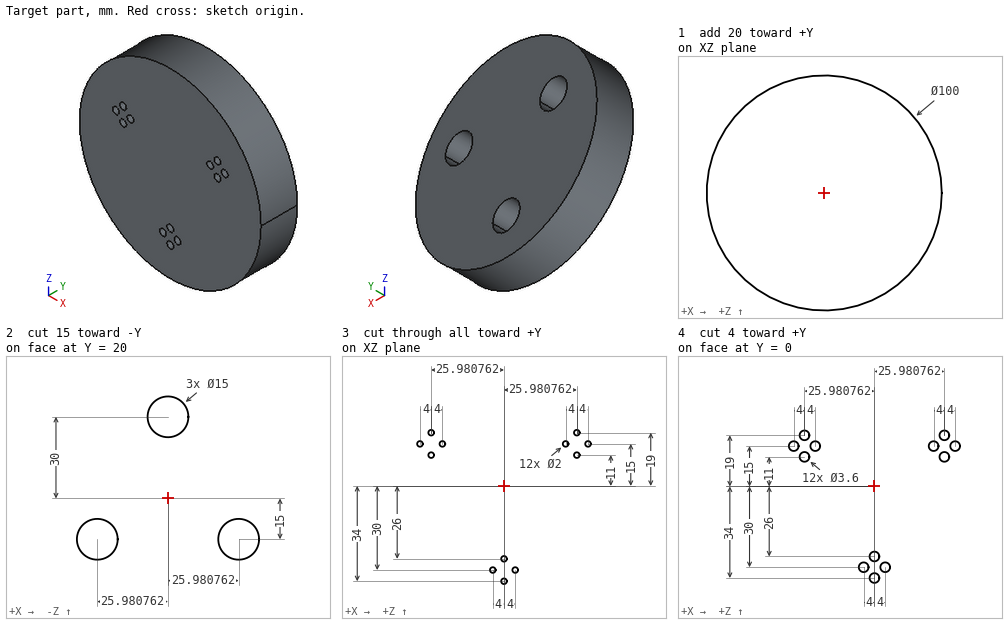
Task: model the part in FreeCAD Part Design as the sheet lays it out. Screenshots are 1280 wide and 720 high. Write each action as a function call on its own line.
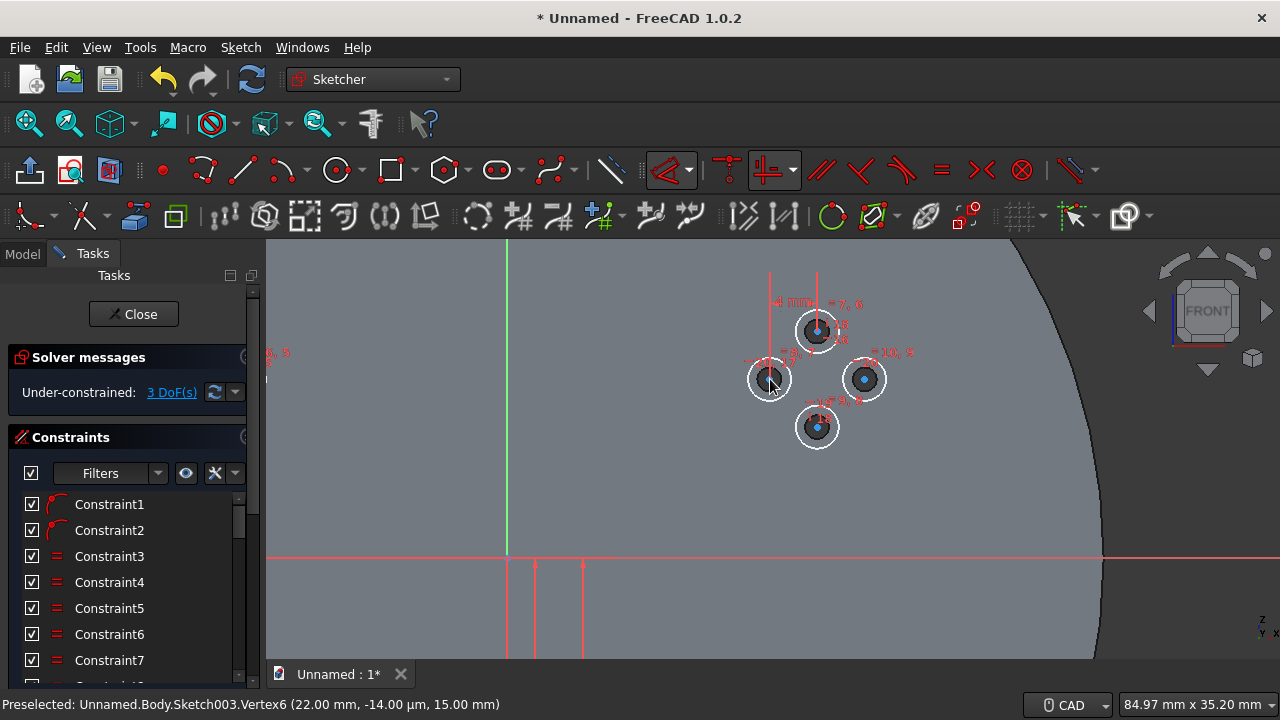
click(817, 332)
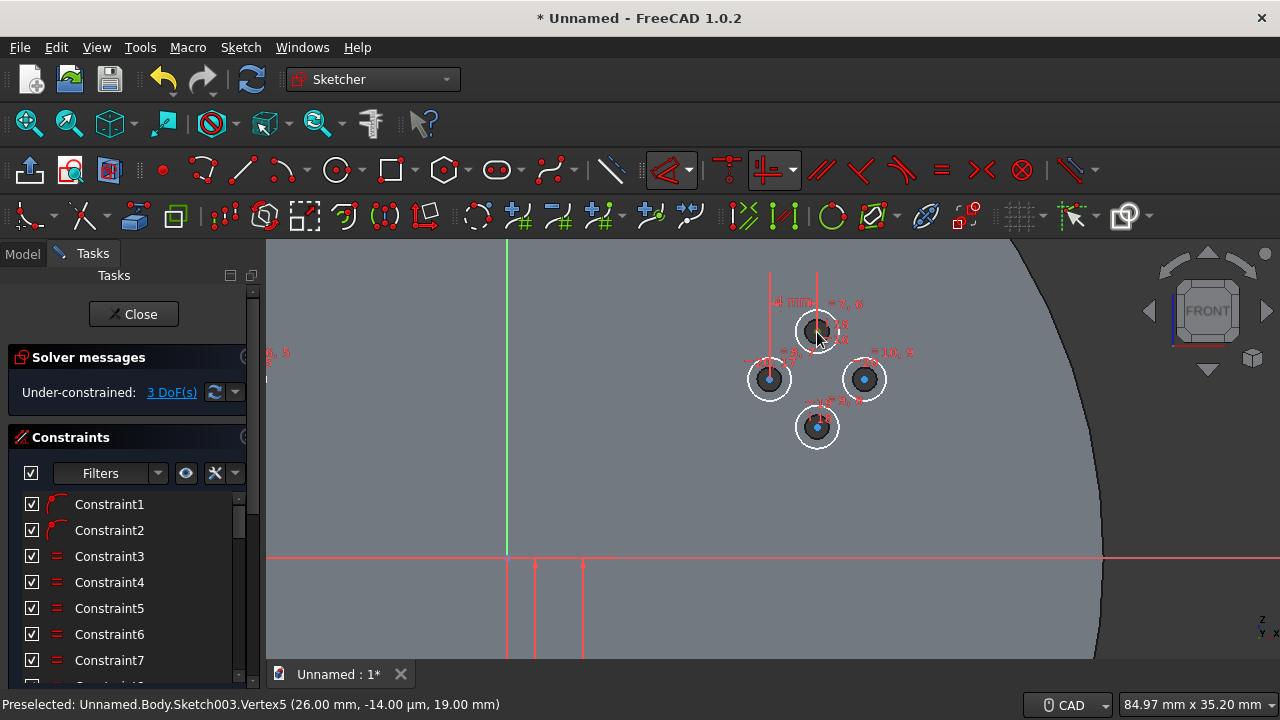
click(865, 379)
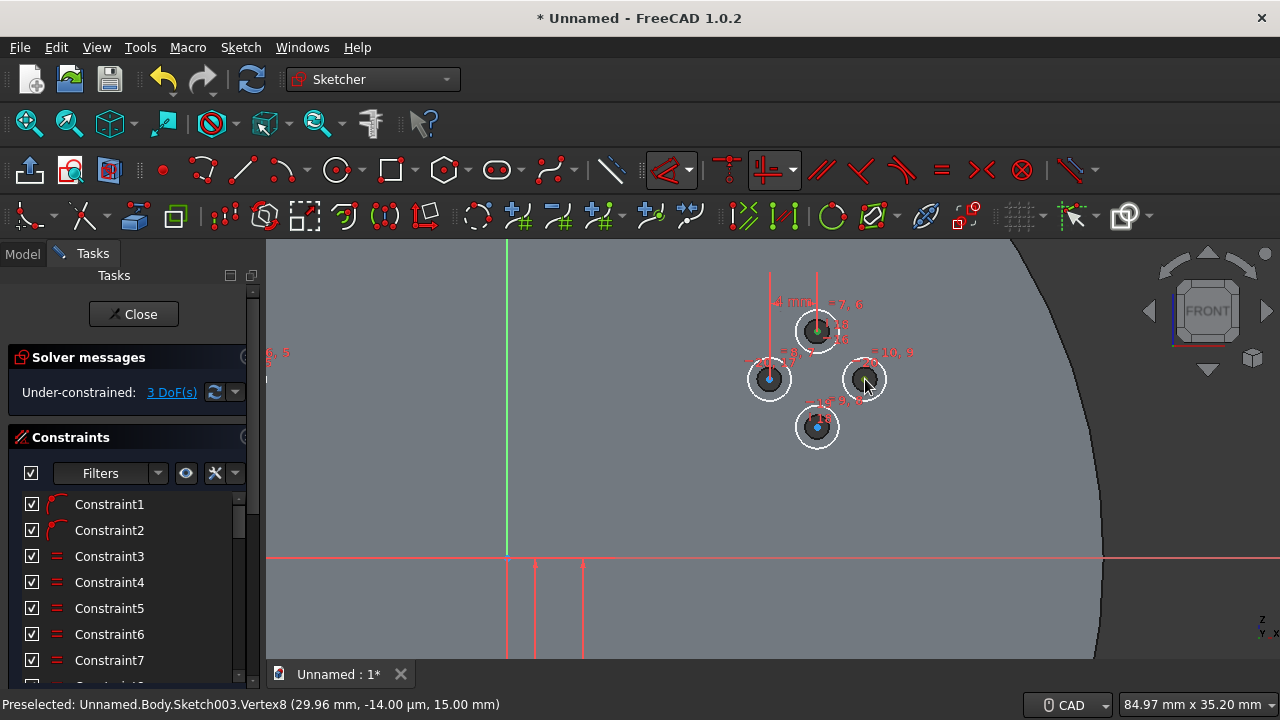
click(692, 170)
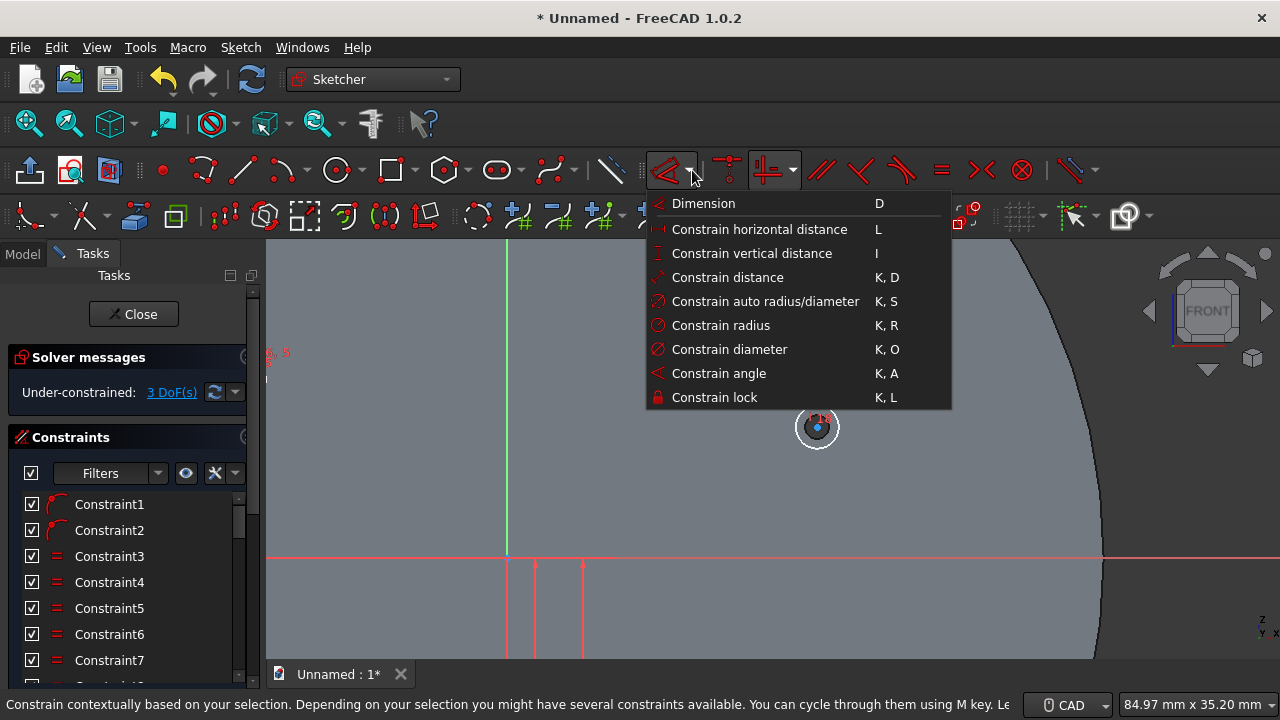
click(799, 229)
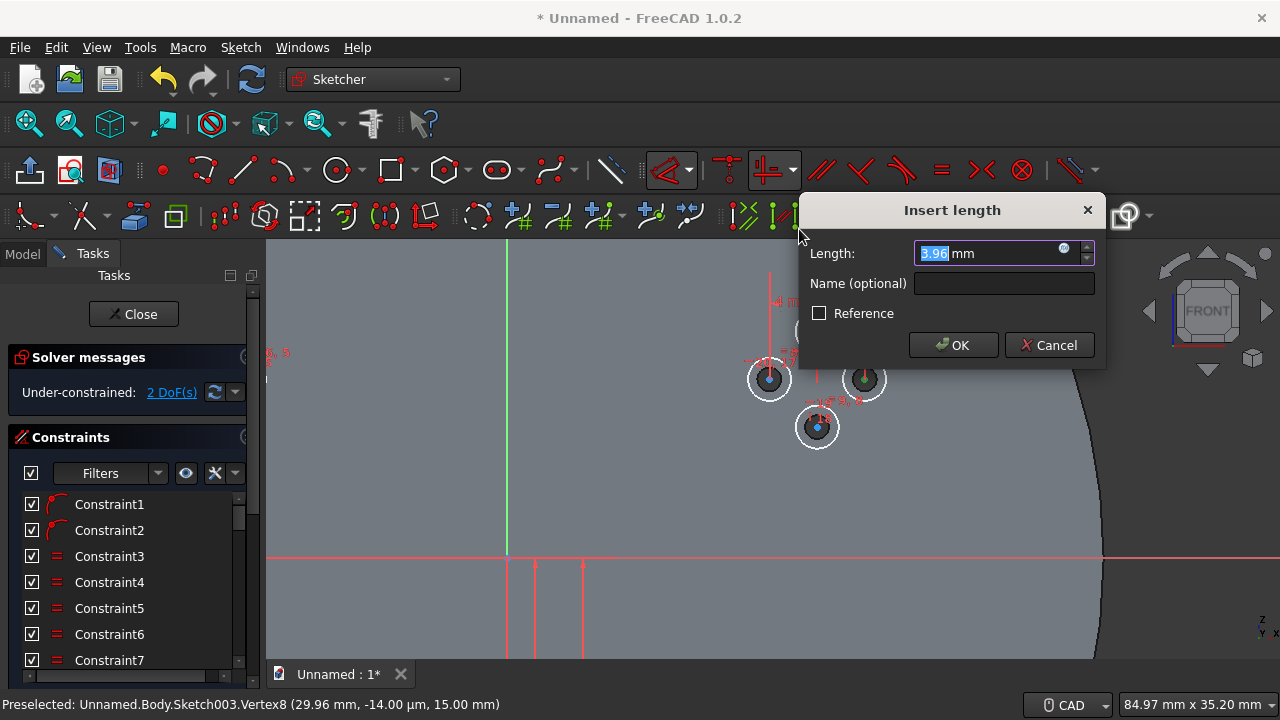
text(4)
key(Return)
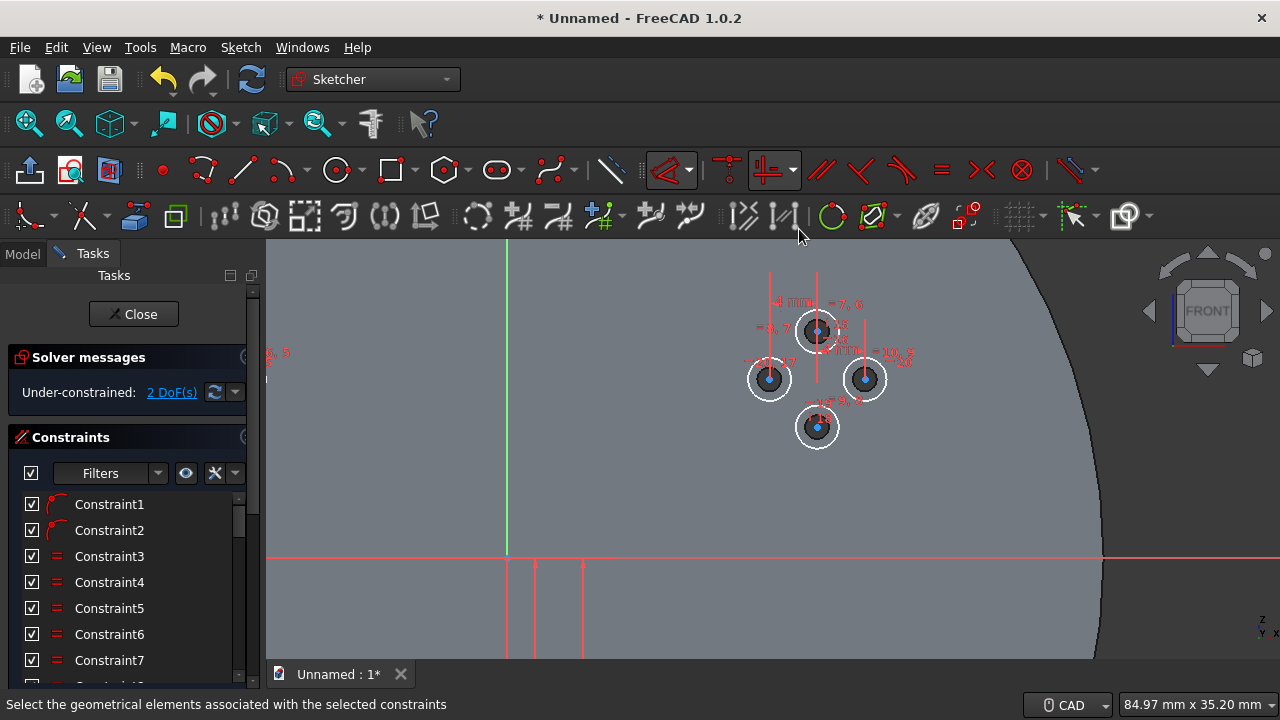
scroll(819, 333, down, 5)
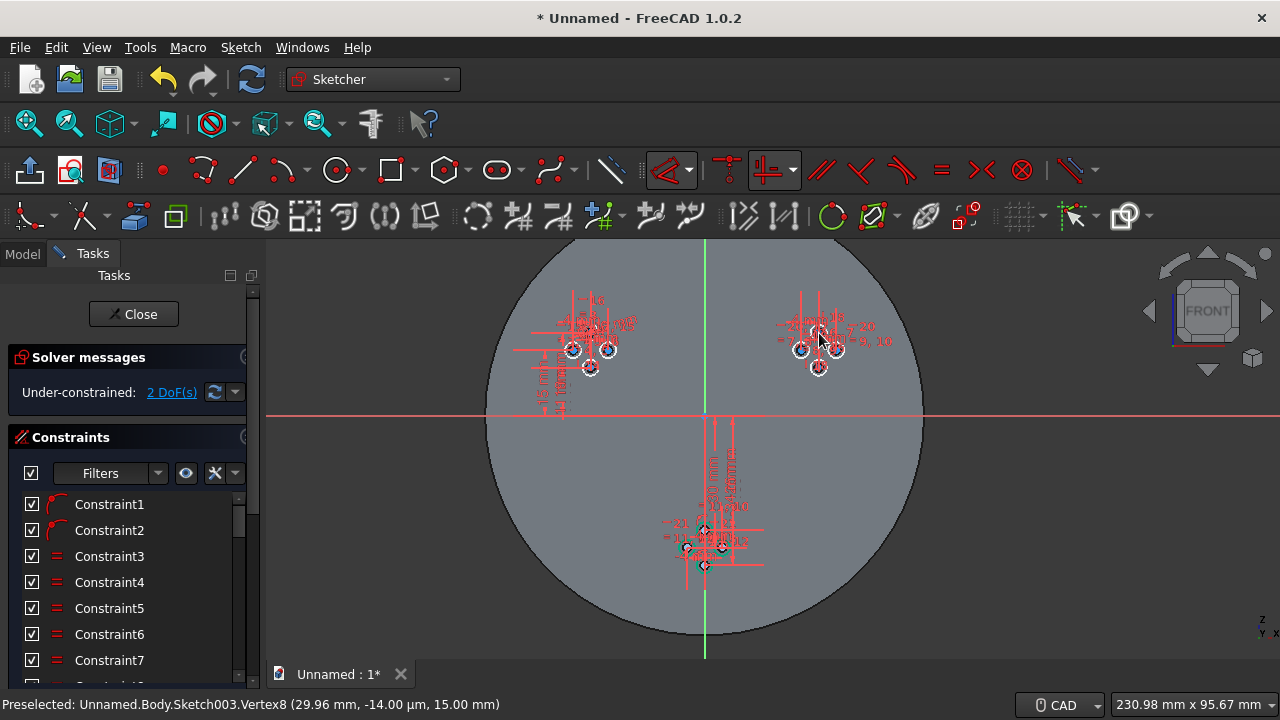
click(591, 333)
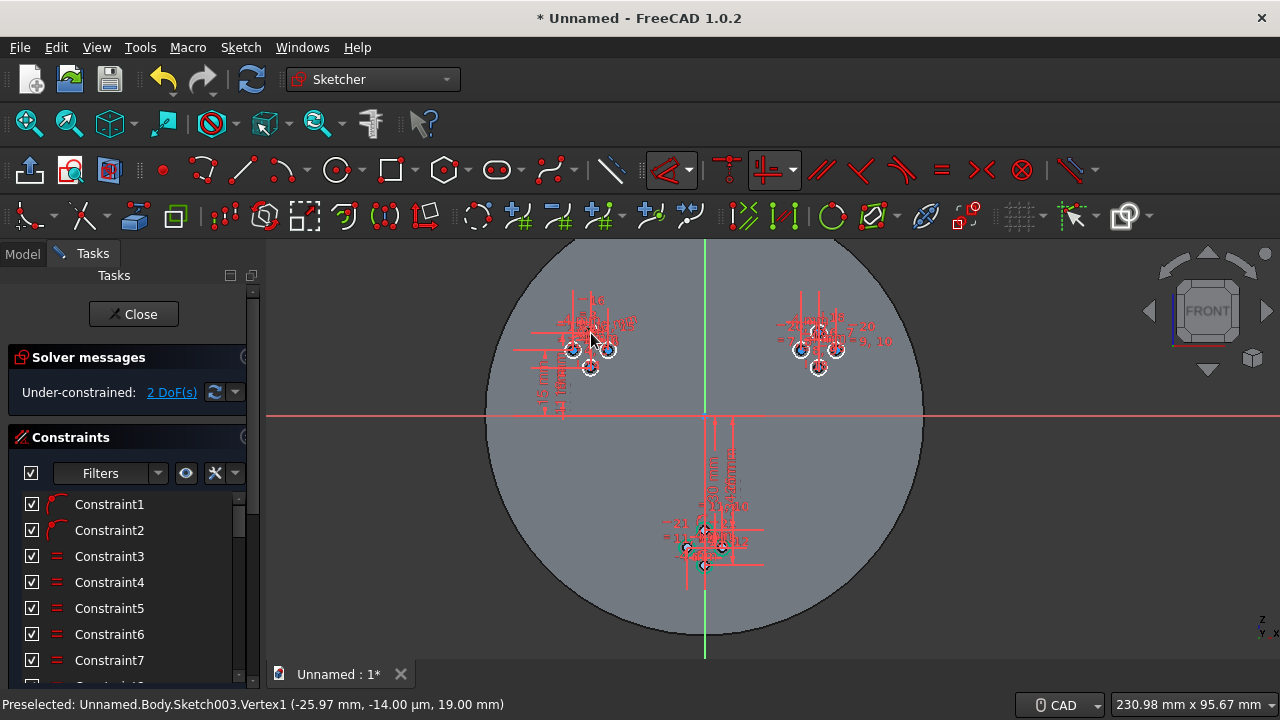
key(l)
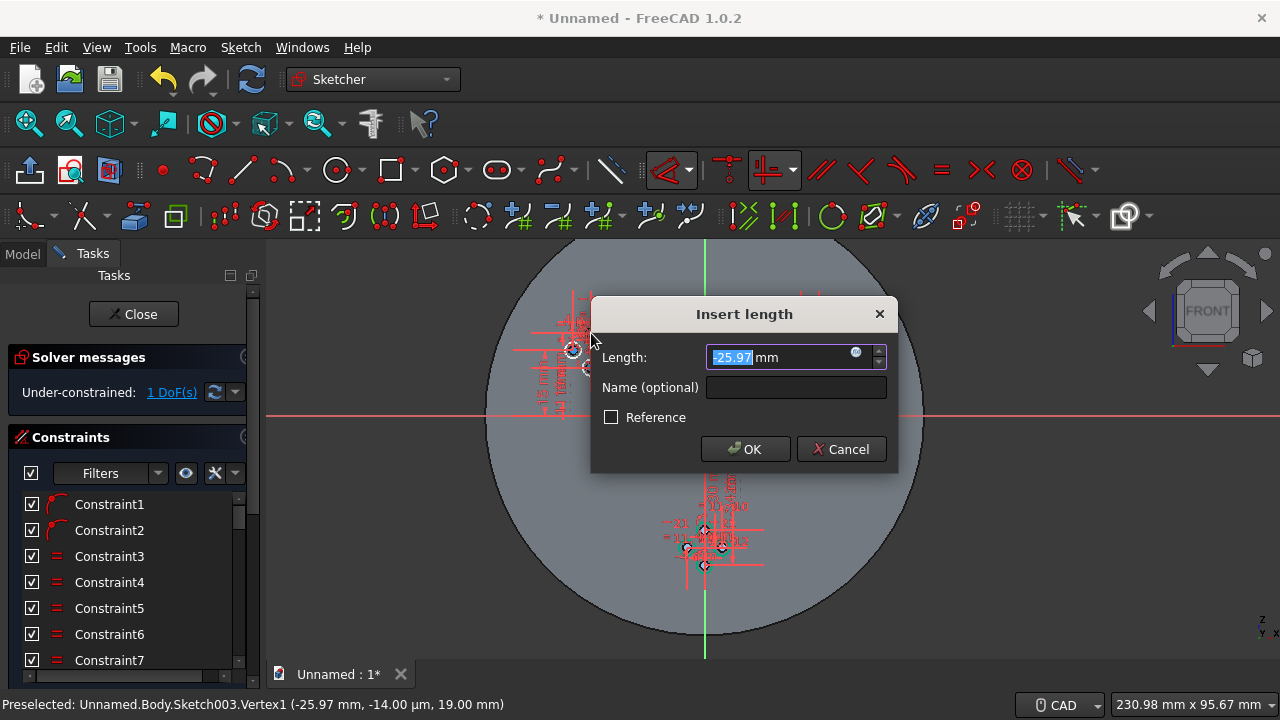
text(-25.980762)
key(Return)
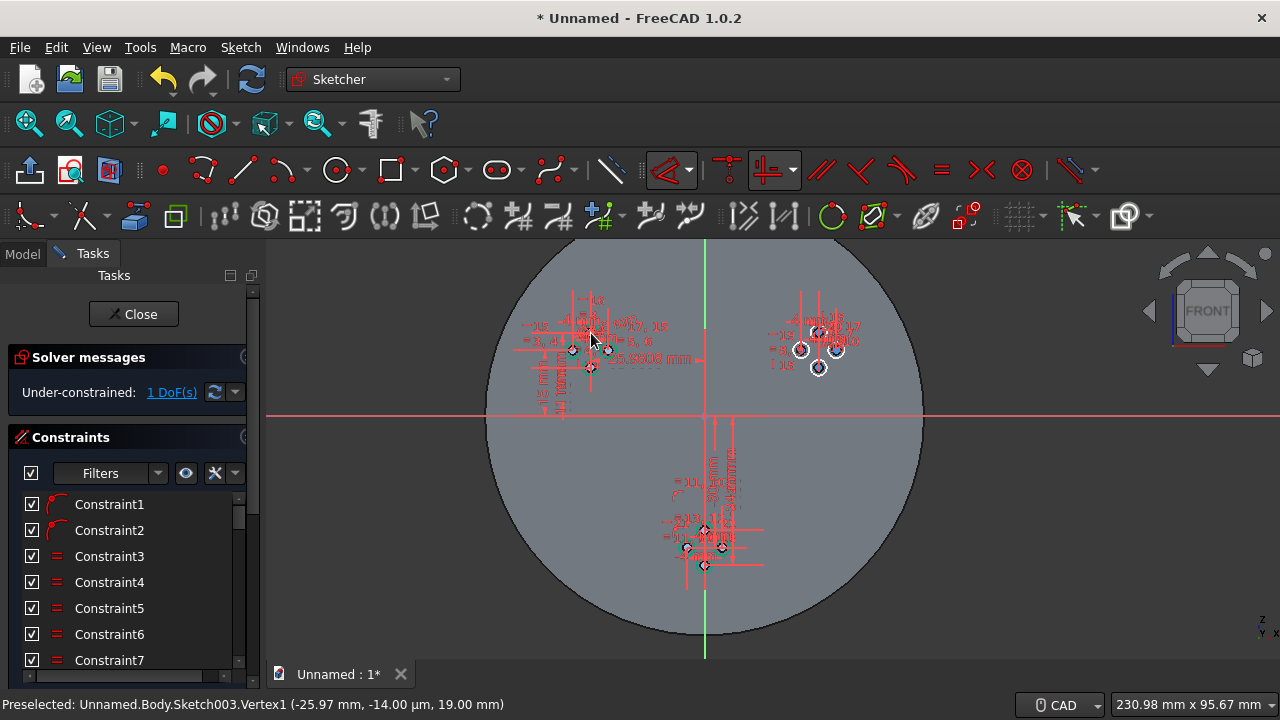
scroll(819, 333, up, 4)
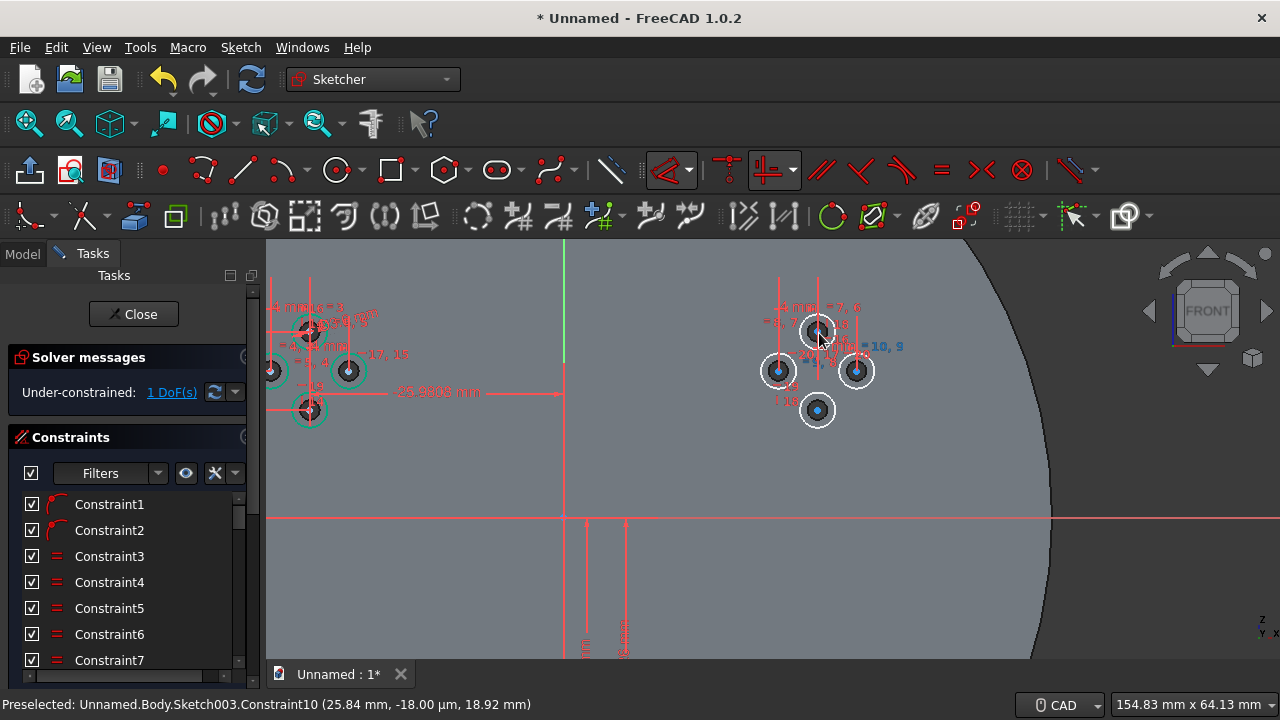
click(818, 332)